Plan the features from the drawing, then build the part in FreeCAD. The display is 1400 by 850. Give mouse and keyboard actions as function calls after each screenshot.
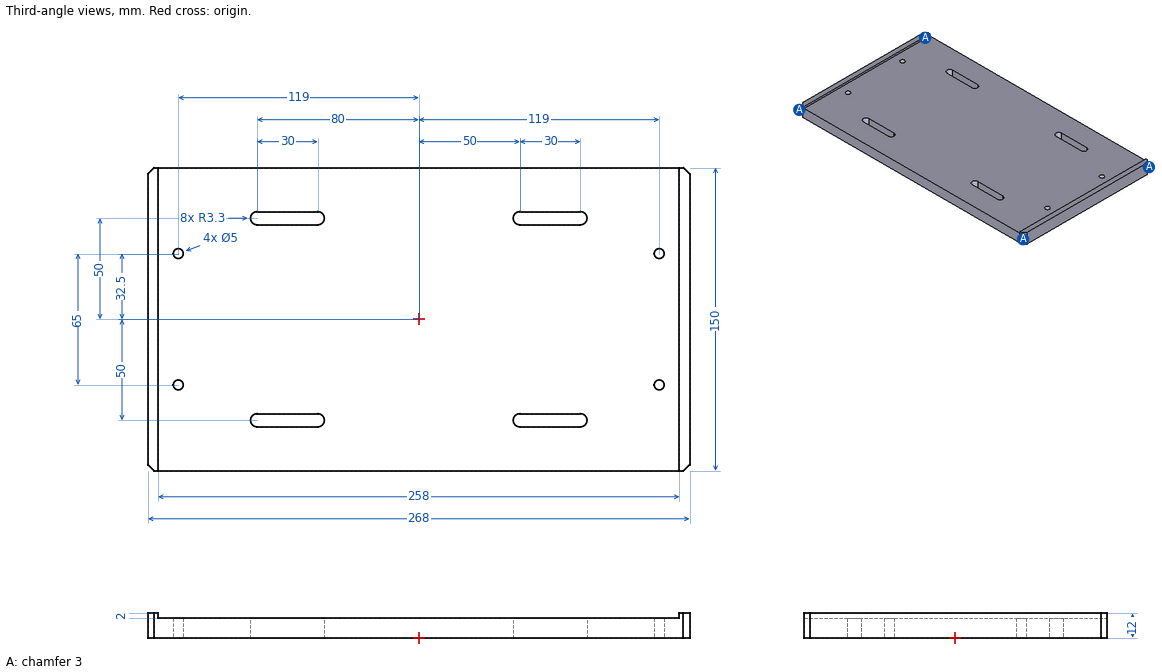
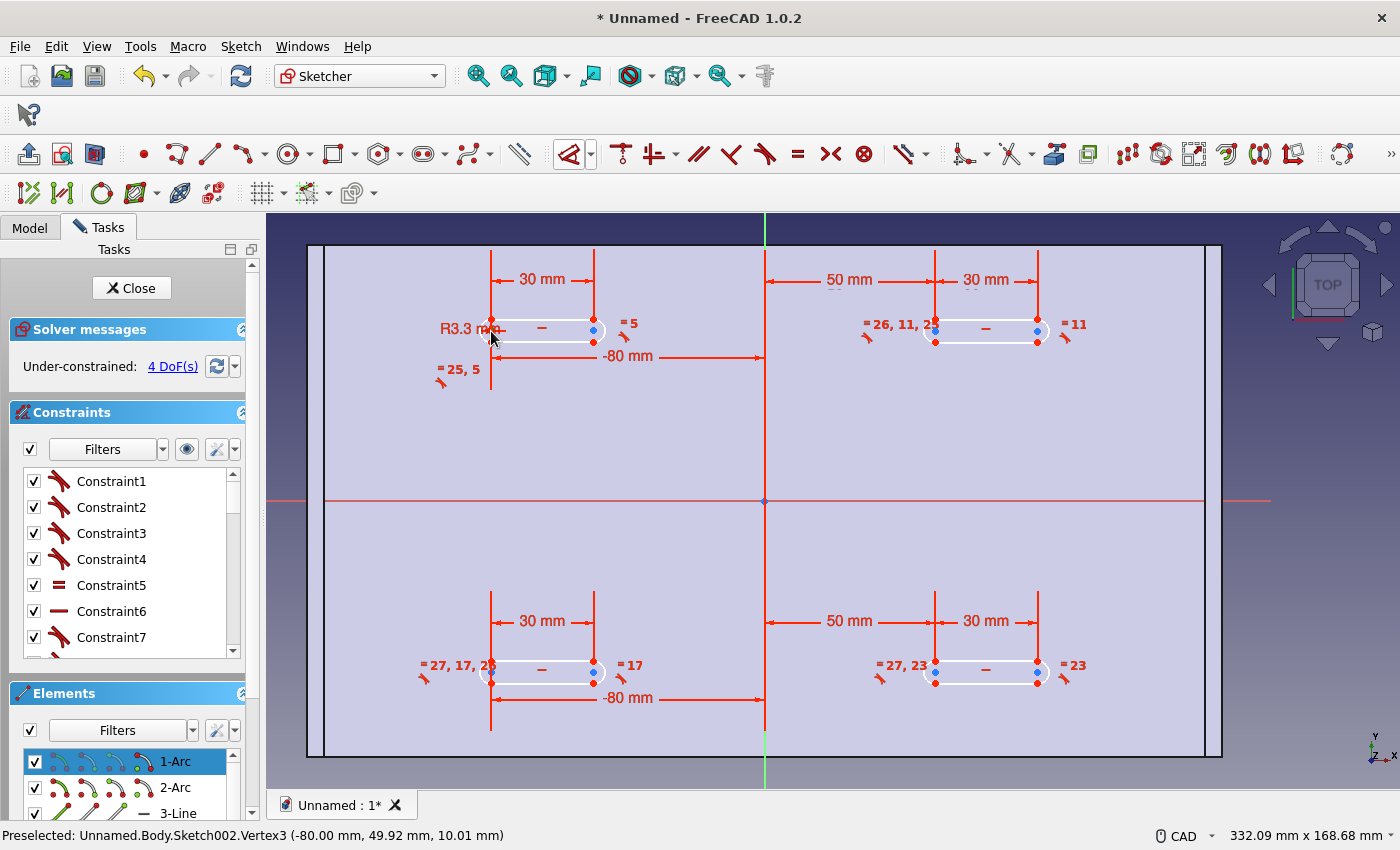
key(i)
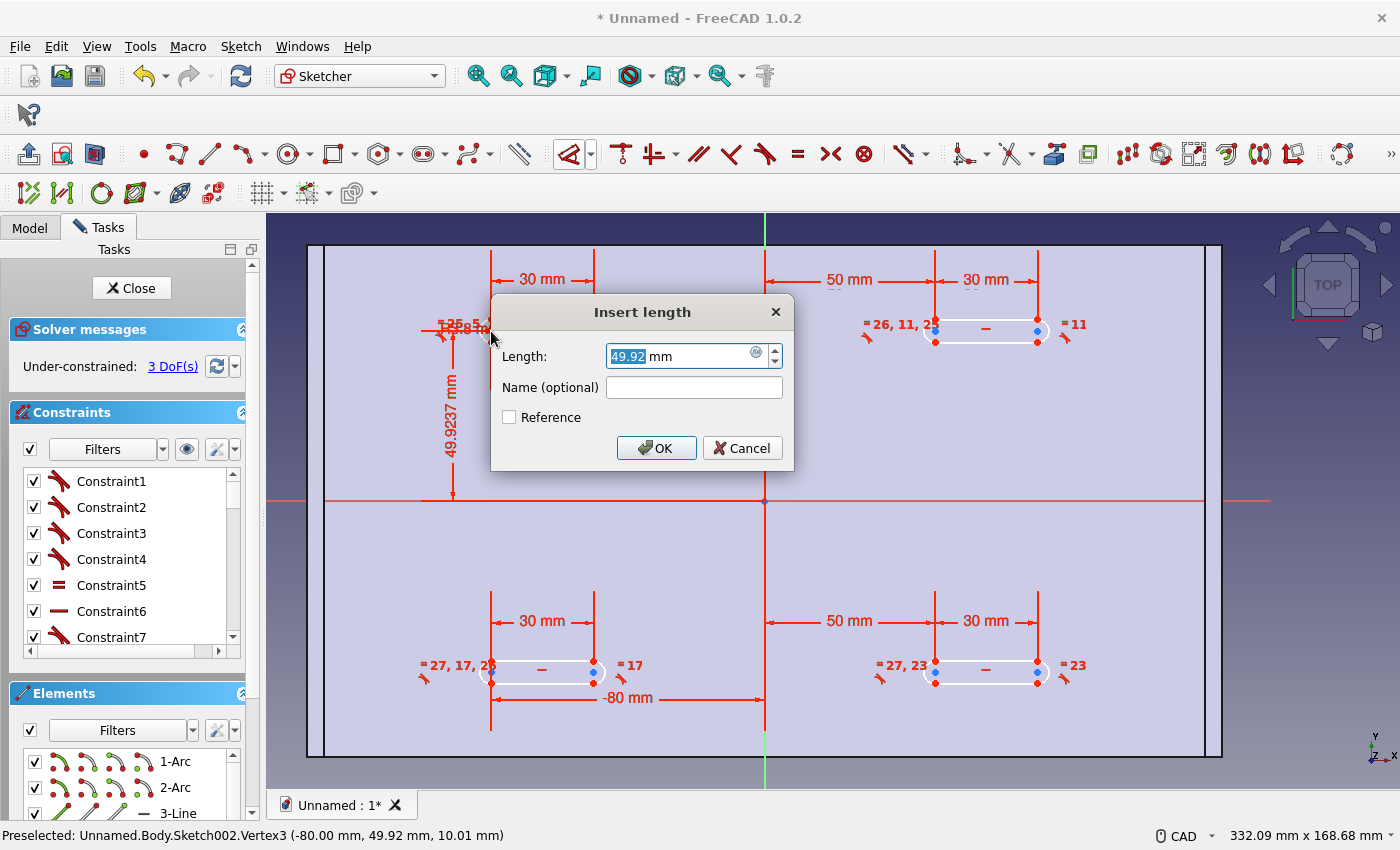
text(50)
key(Return)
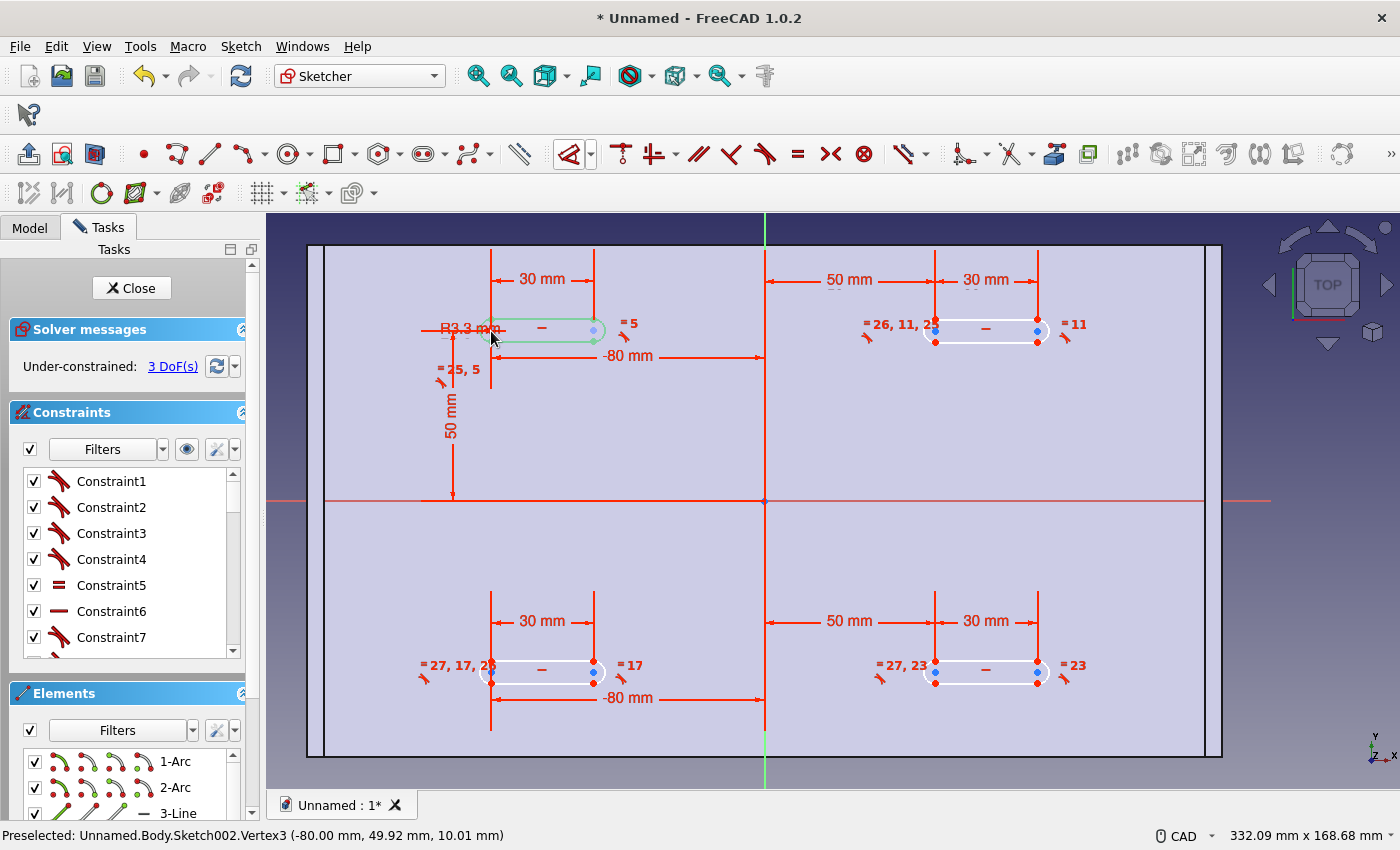
click(935, 331)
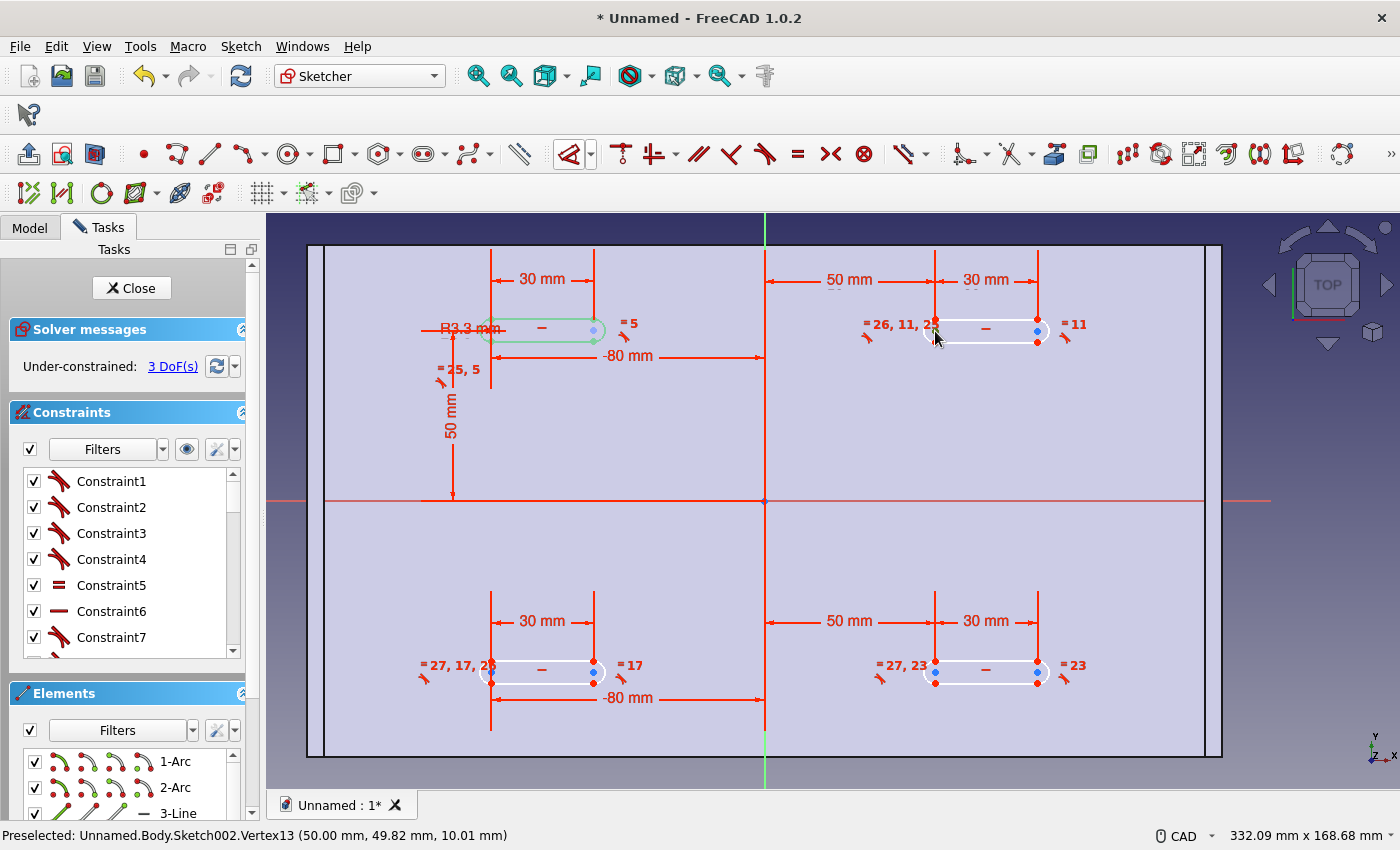
click(590, 154)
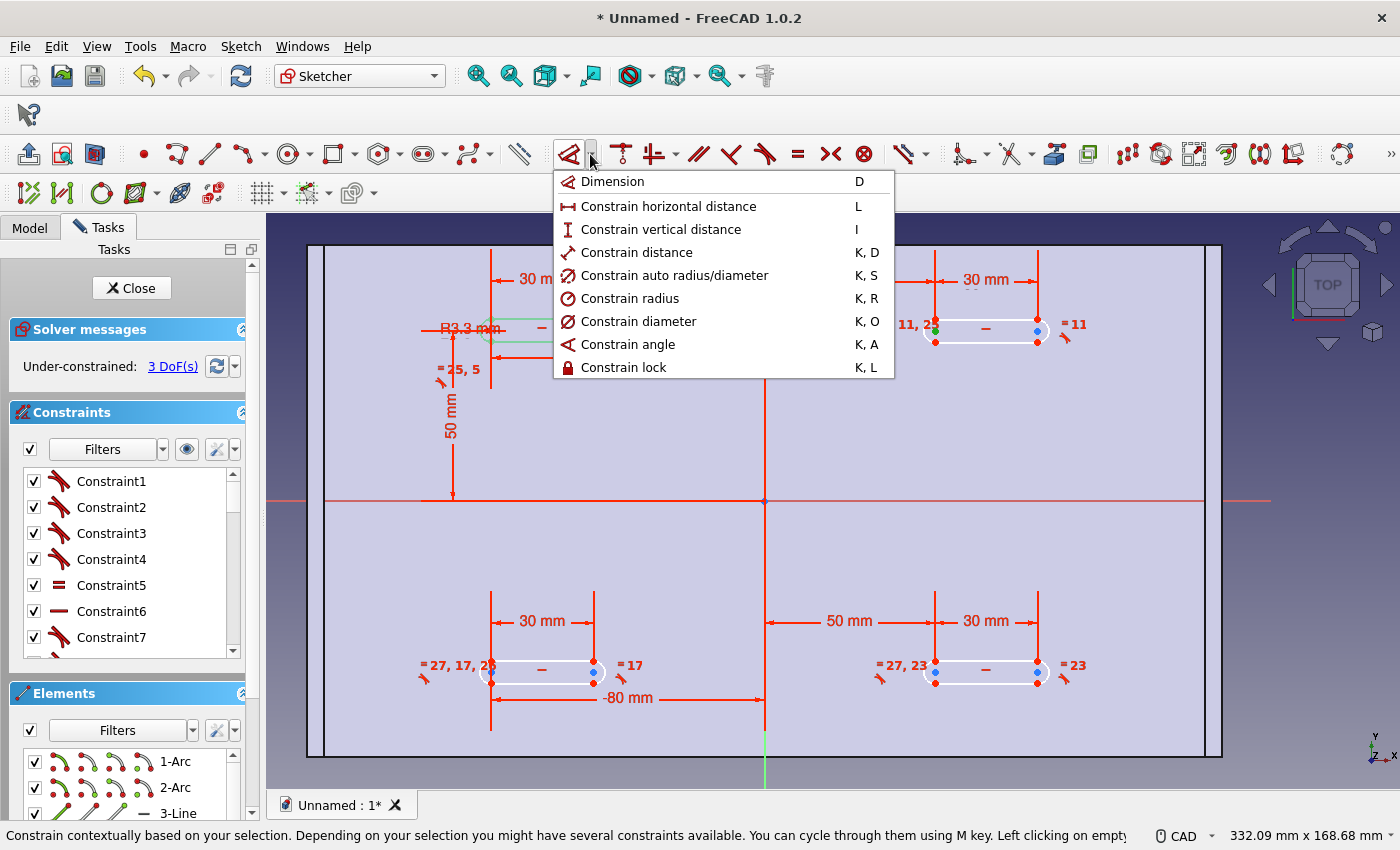
click(724, 230)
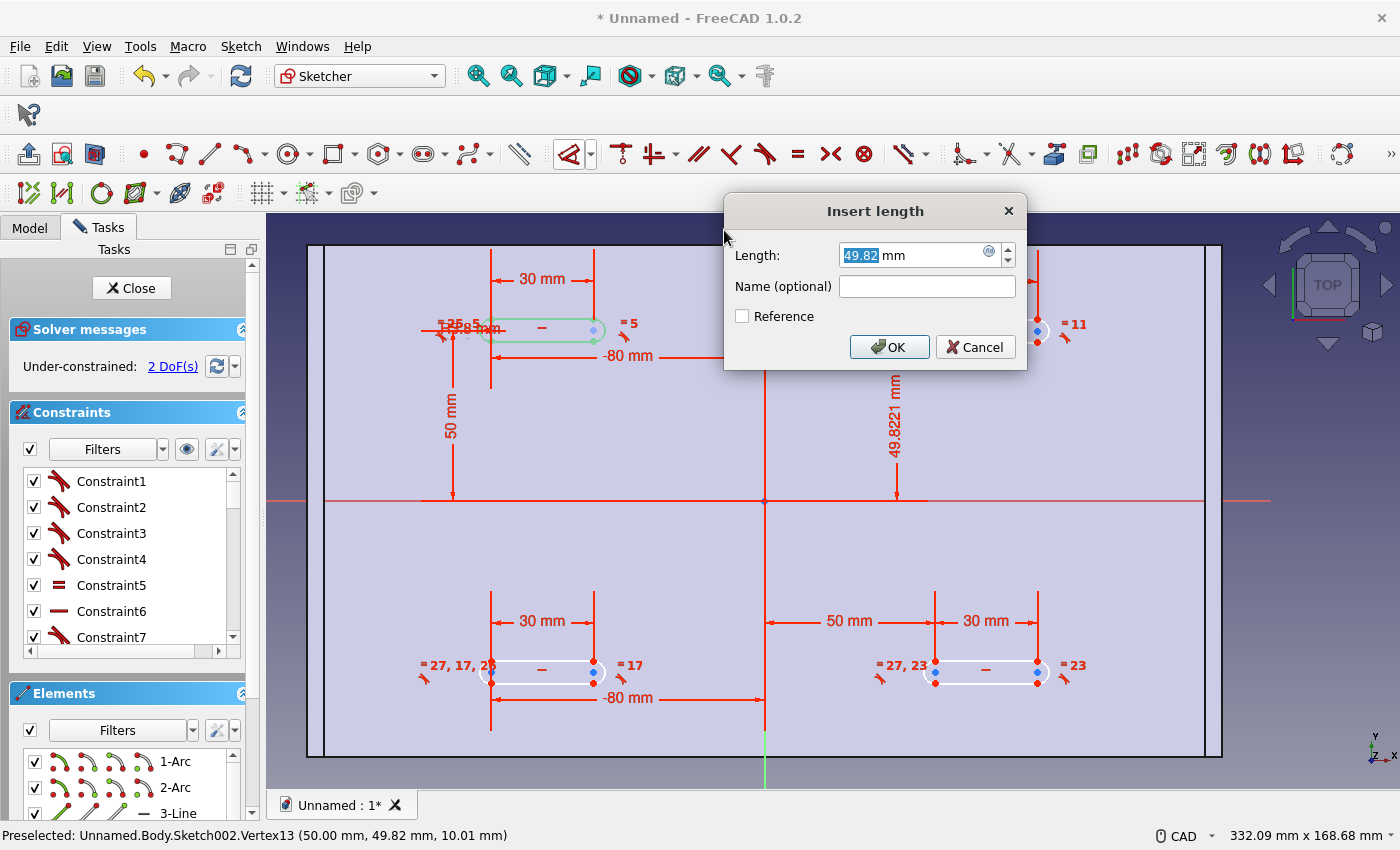
text(50)
key(Return)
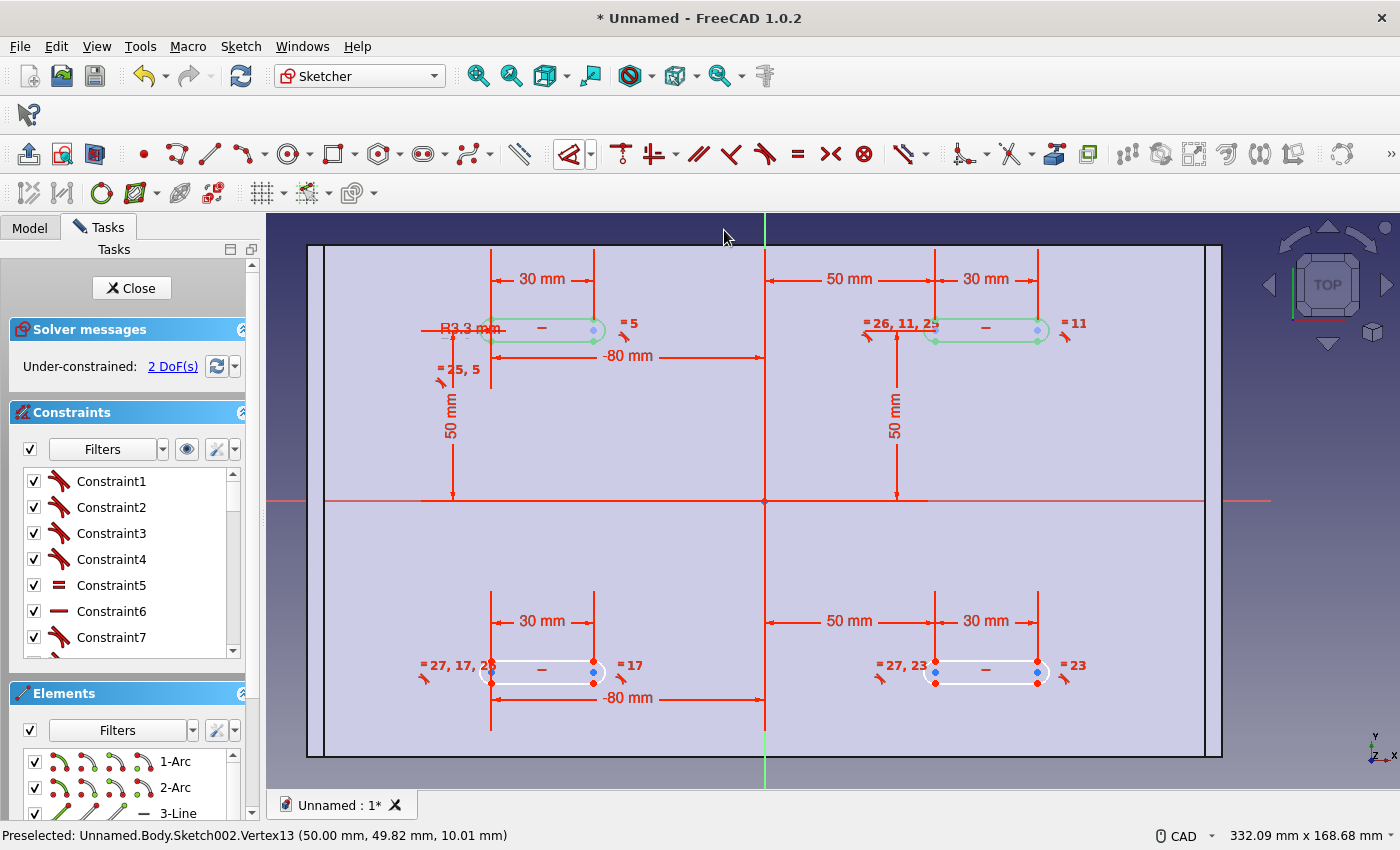
click(491, 673)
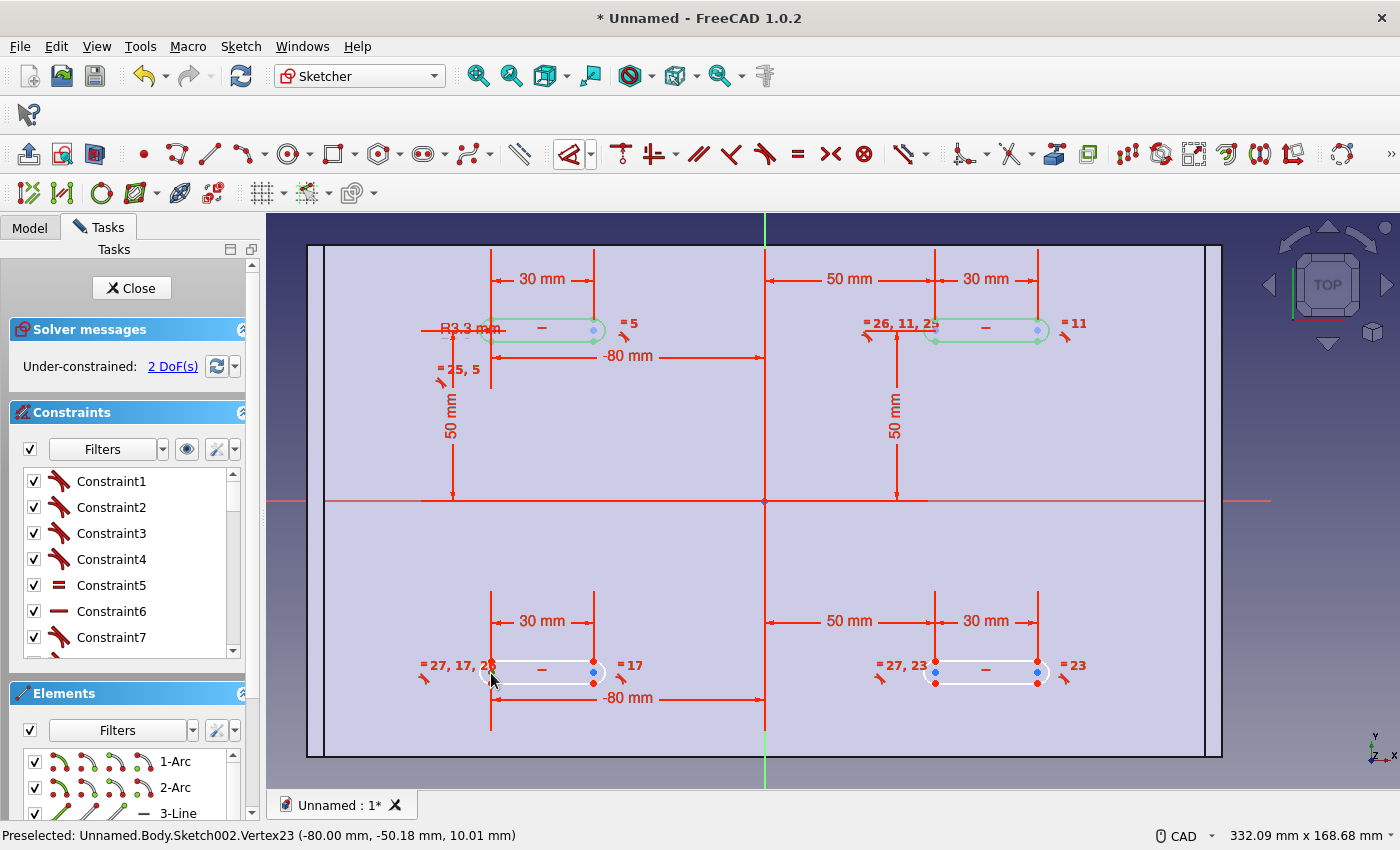
key(i)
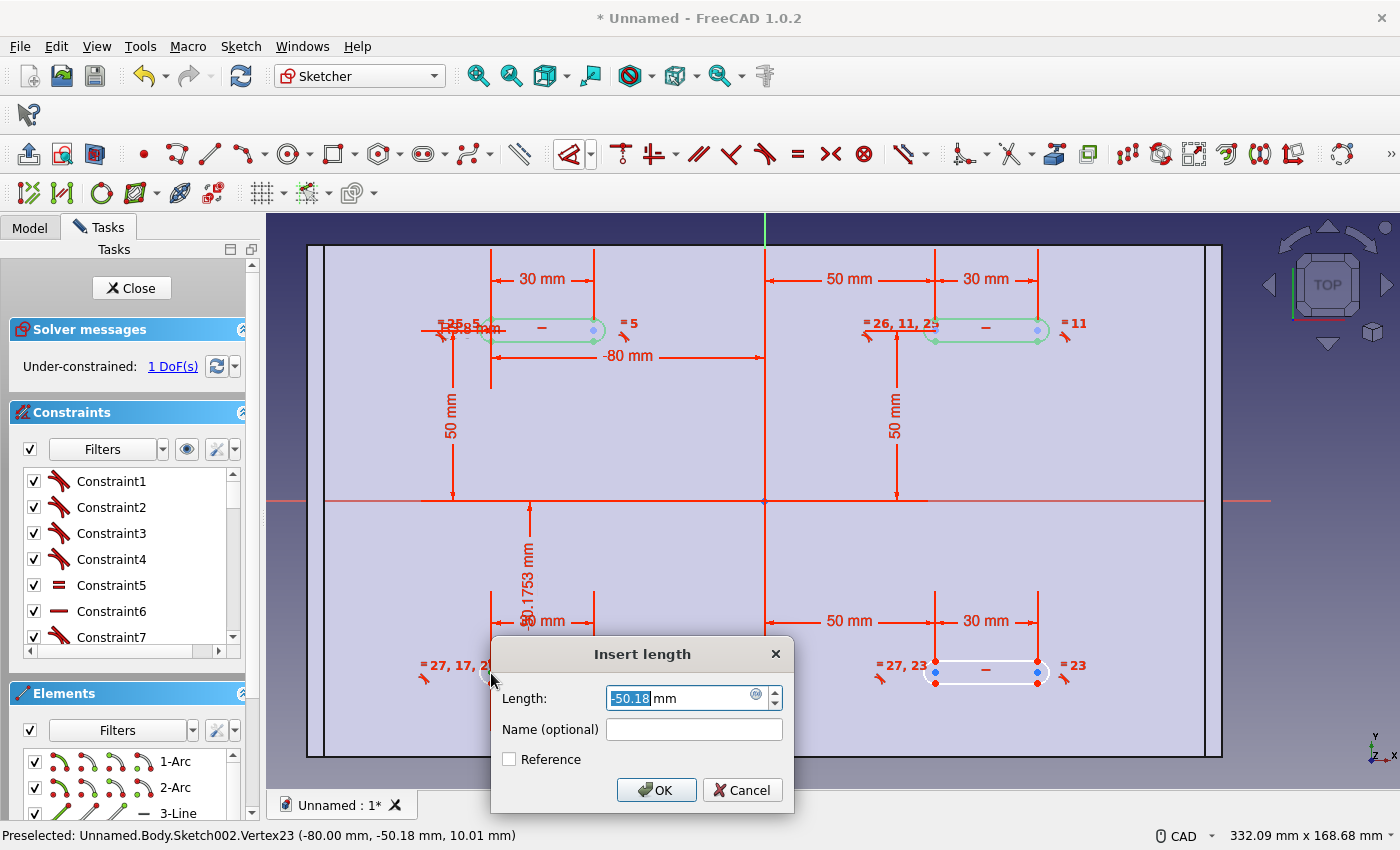
text(-50)
key(Return)